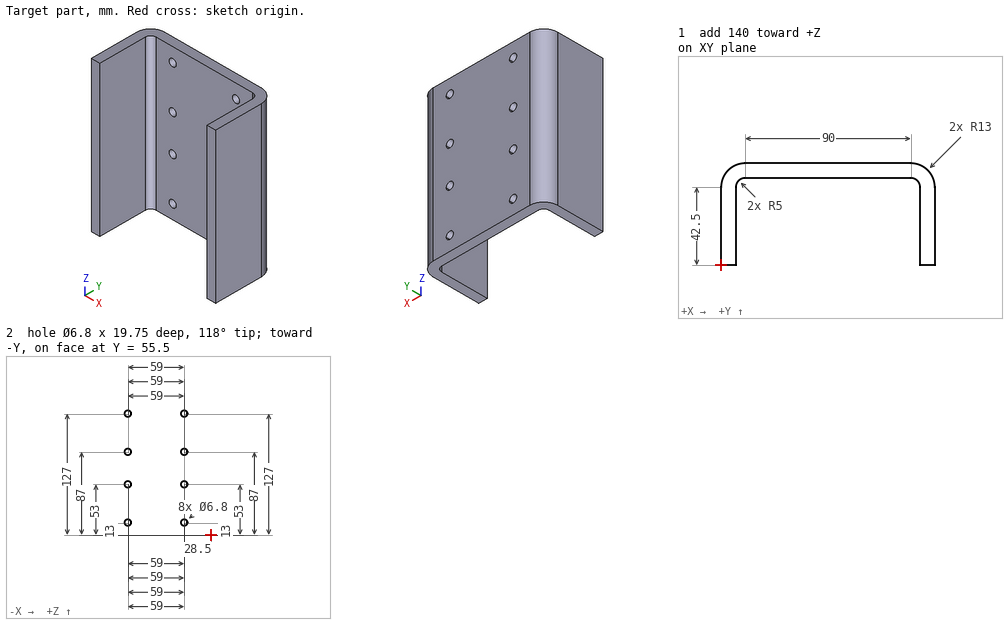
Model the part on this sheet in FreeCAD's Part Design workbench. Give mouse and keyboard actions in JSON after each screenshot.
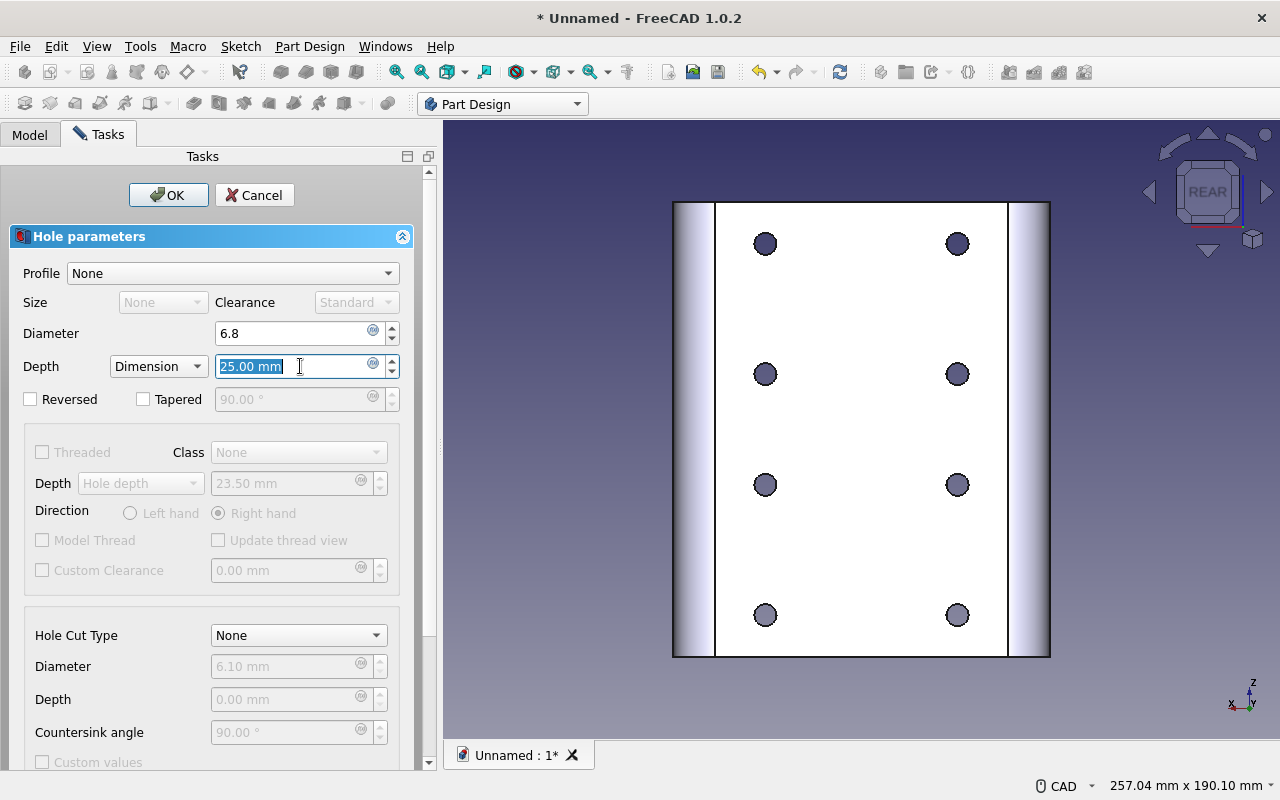
{"action": "type", "text": "19.75"}
{"action": "key", "text": "Tab"}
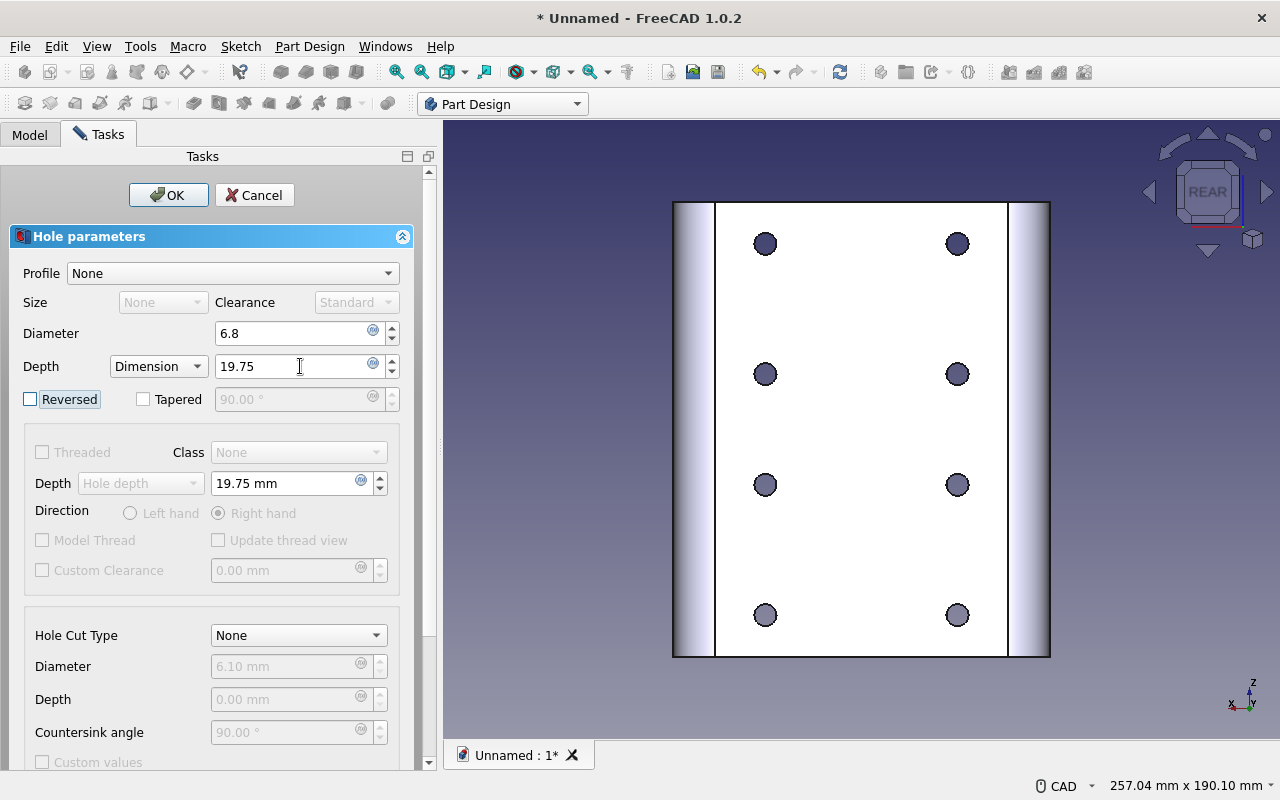
{"action": "left_click", "coordinate": [169, 195]}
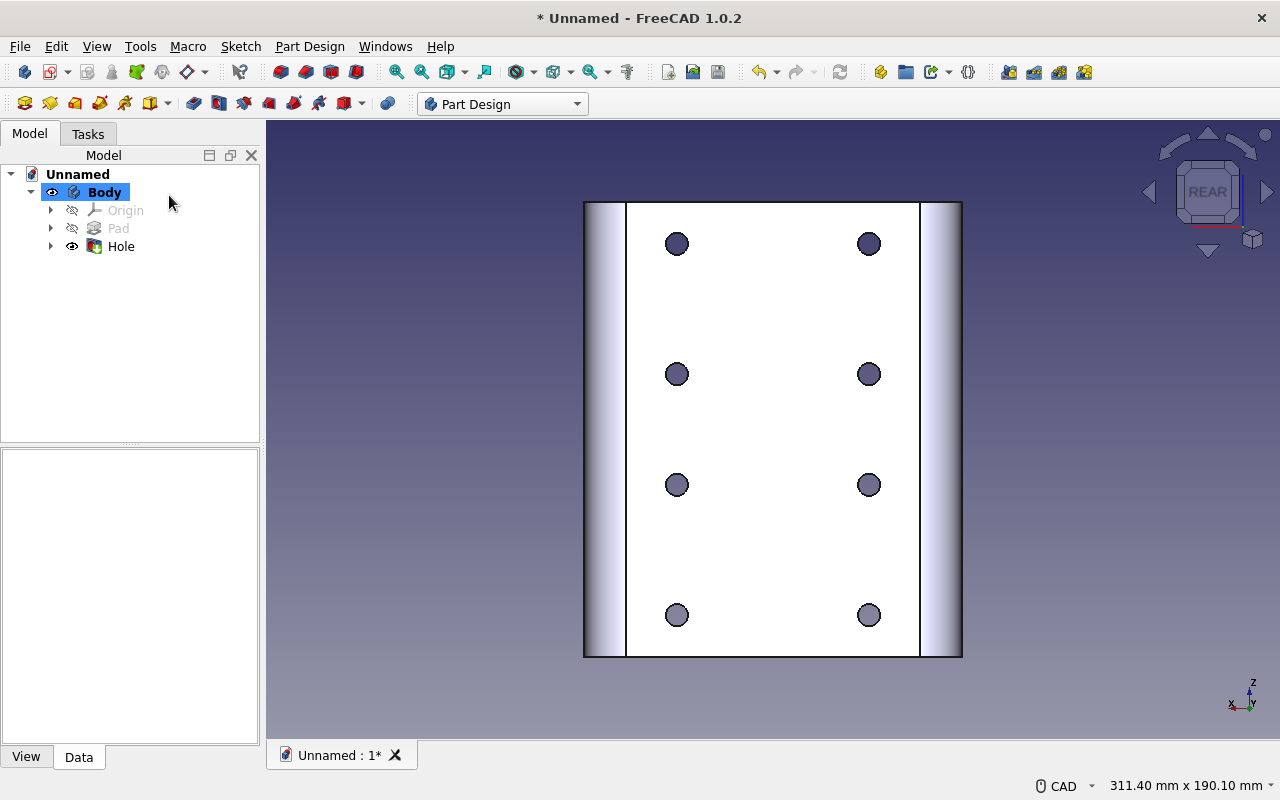
{"action": "key", "text": "0"}